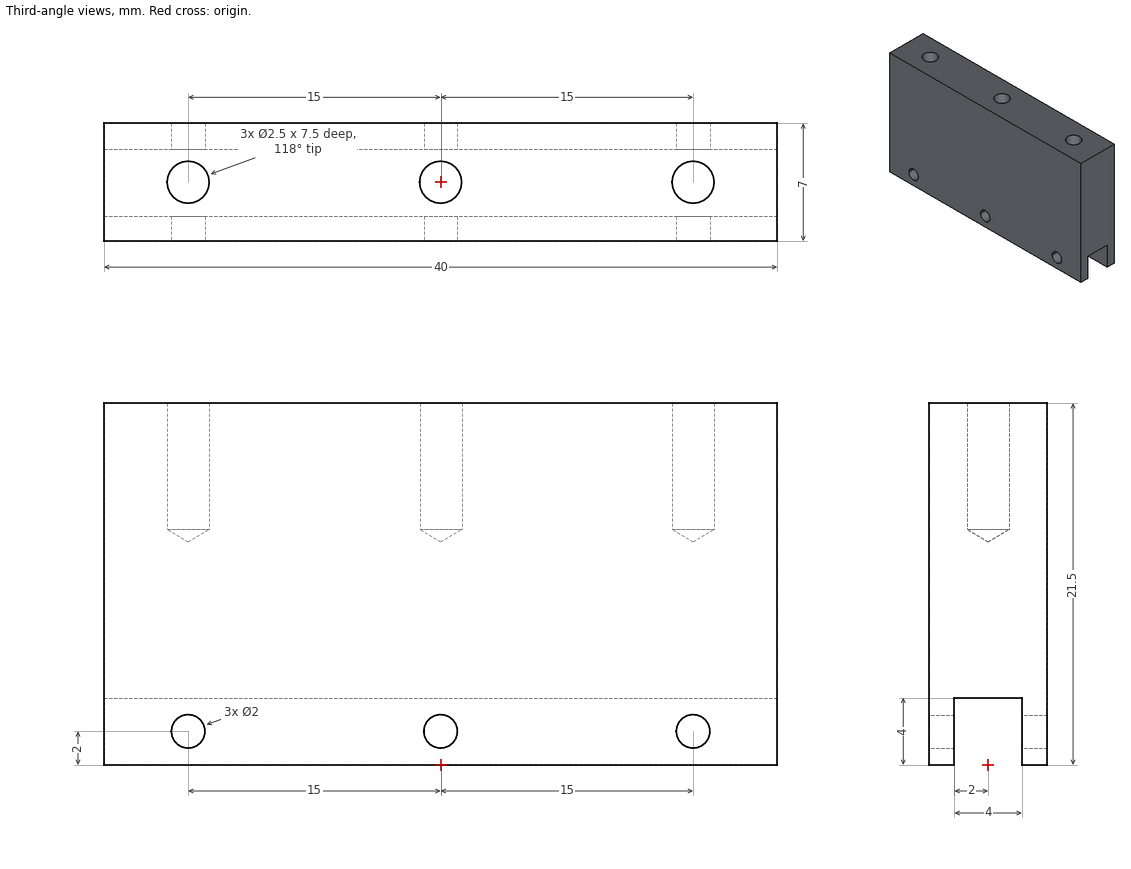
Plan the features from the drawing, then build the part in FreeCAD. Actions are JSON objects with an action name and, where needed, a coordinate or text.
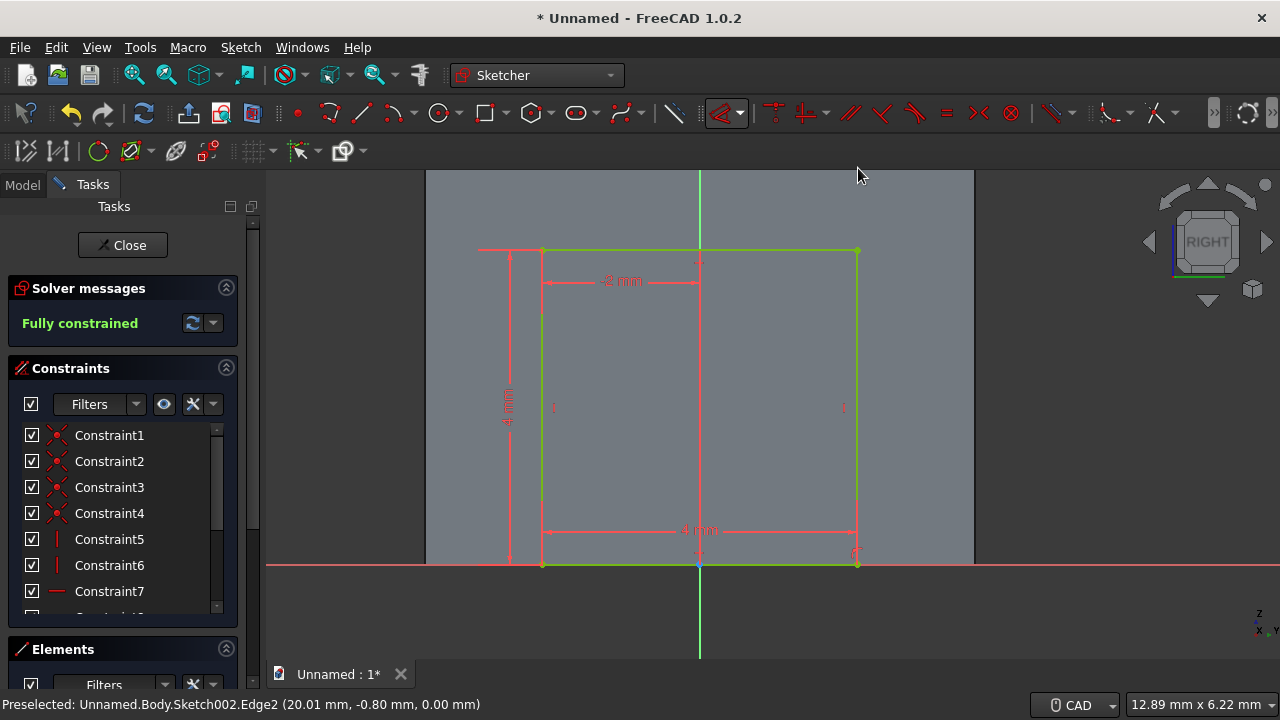
{"action": "left_click", "coordinate": [123, 245]}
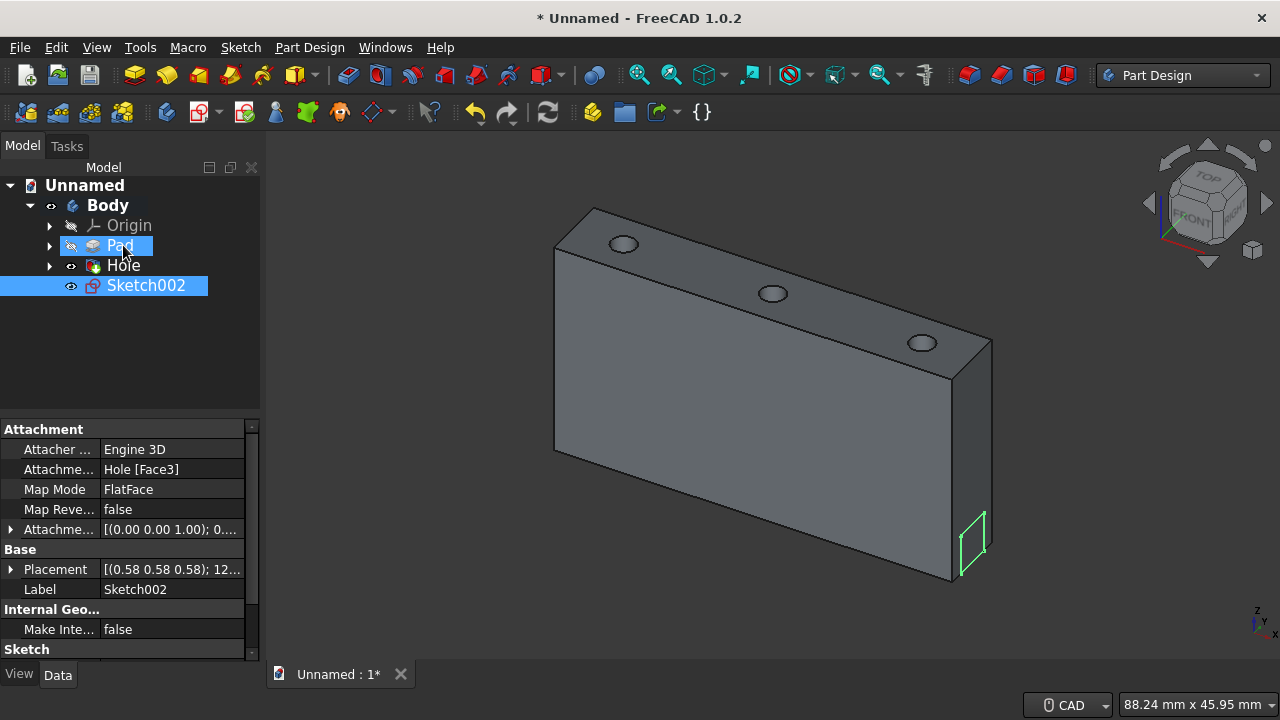
{"action": "left_click", "coordinate": [350, 76]}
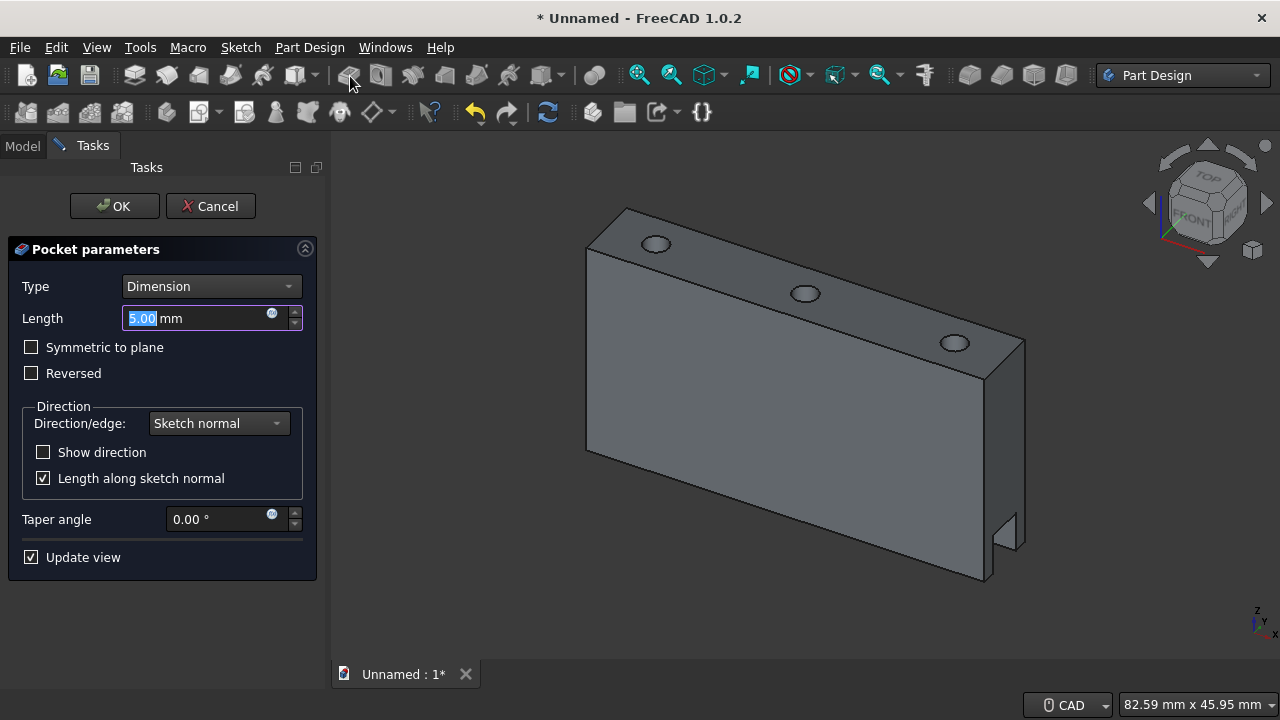
{"action": "left_click", "coordinate": [212, 286]}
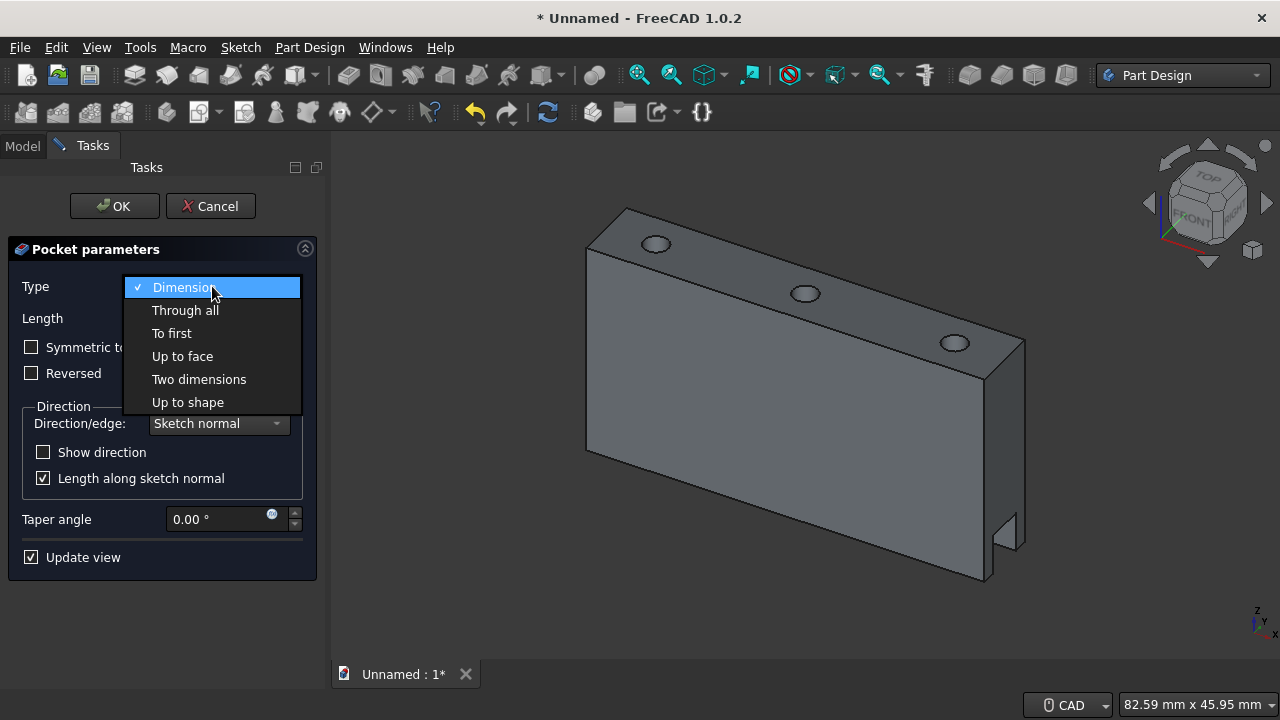
{"action": "left_click", "coordinate": [212, 310]}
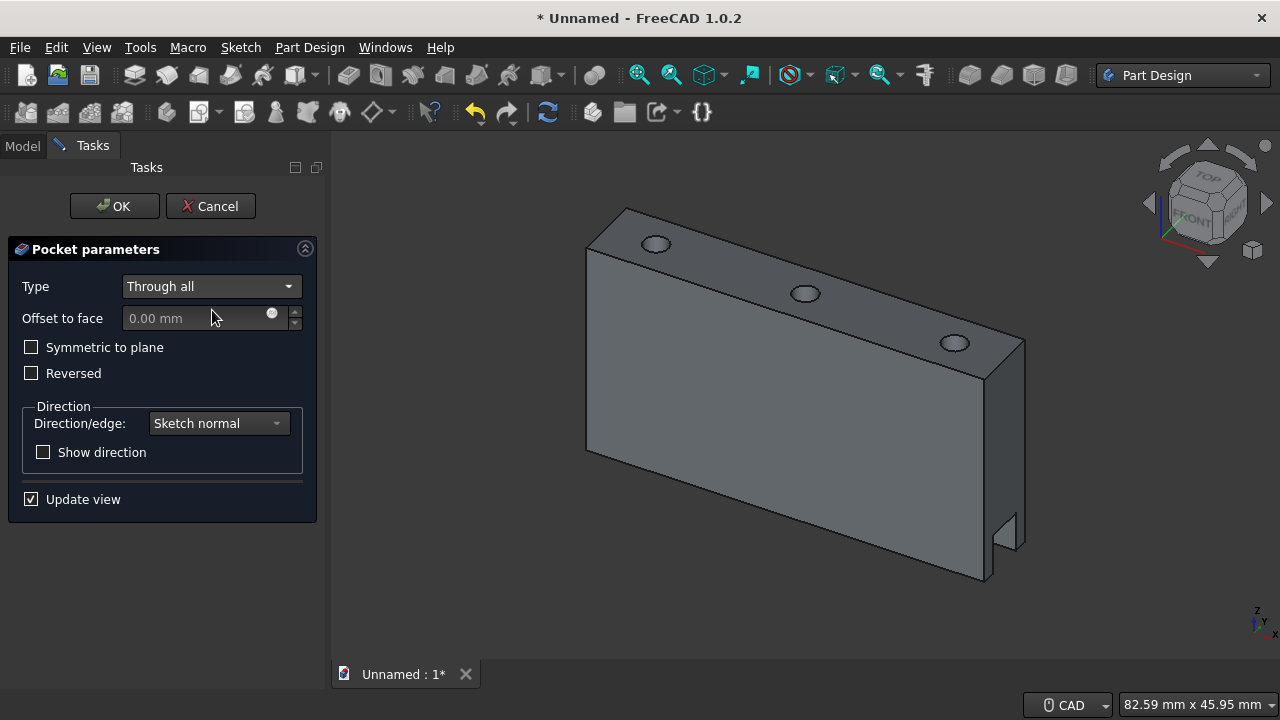
{"action": "left_click", "coordinate": [115, 206]}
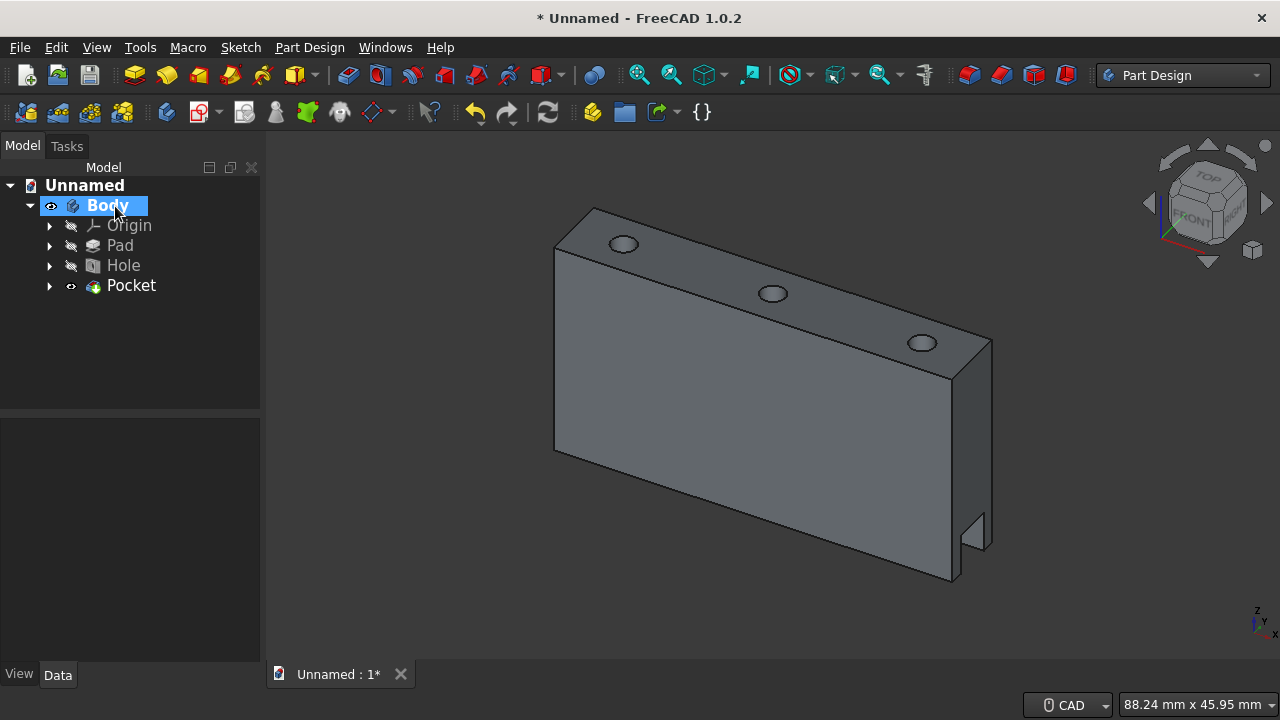
{"action": "key", "text": "4"}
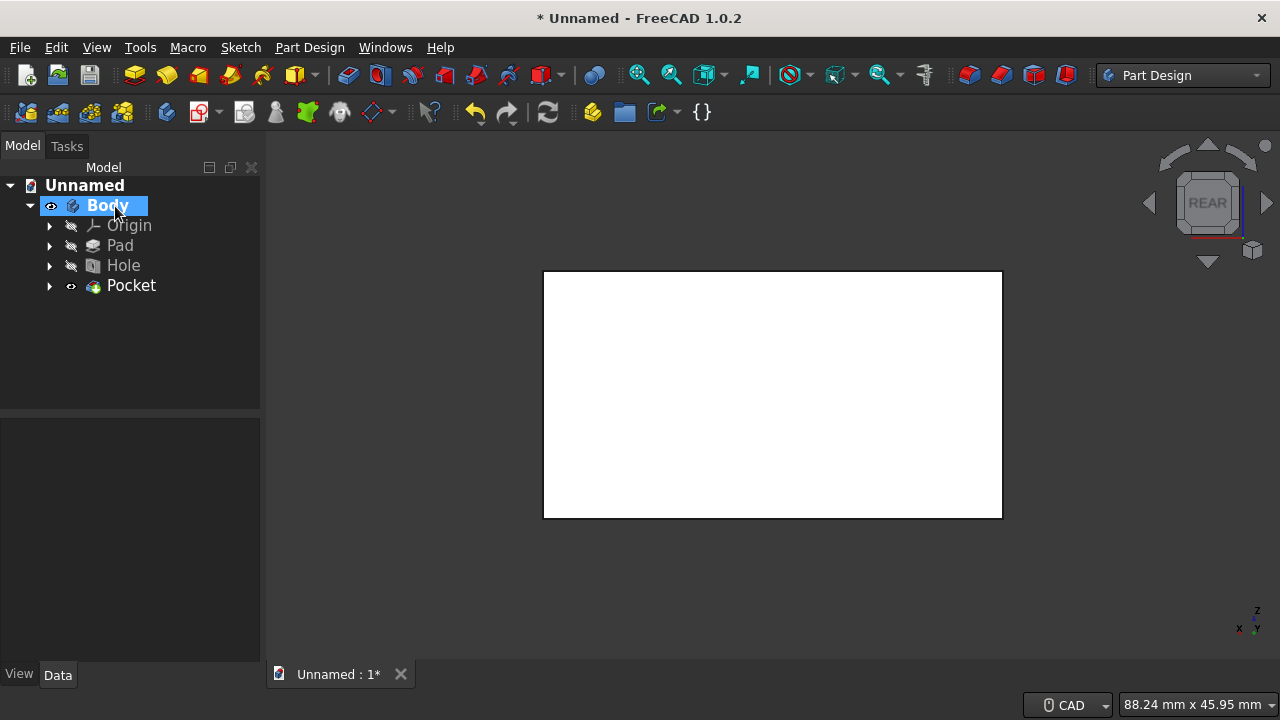
{"action": "left_click", "coordinate": [707, 394]}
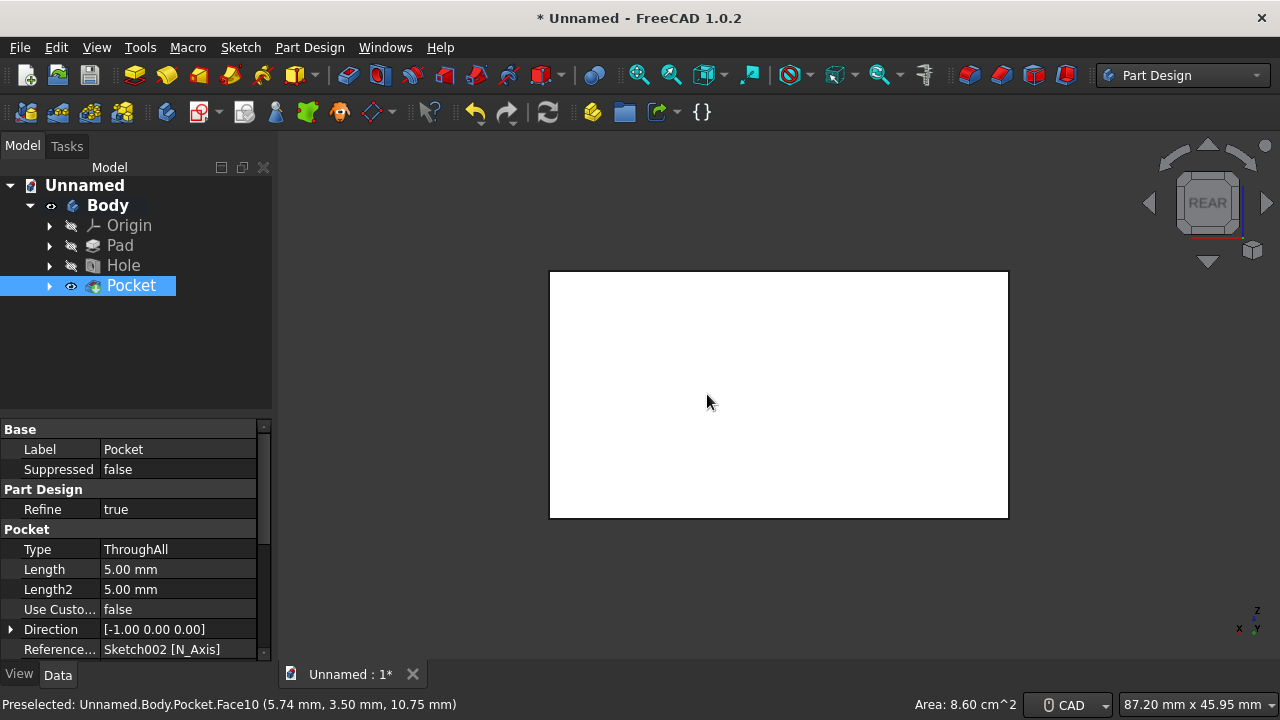
{"action": "left_click", "coordinate": [200, 112]}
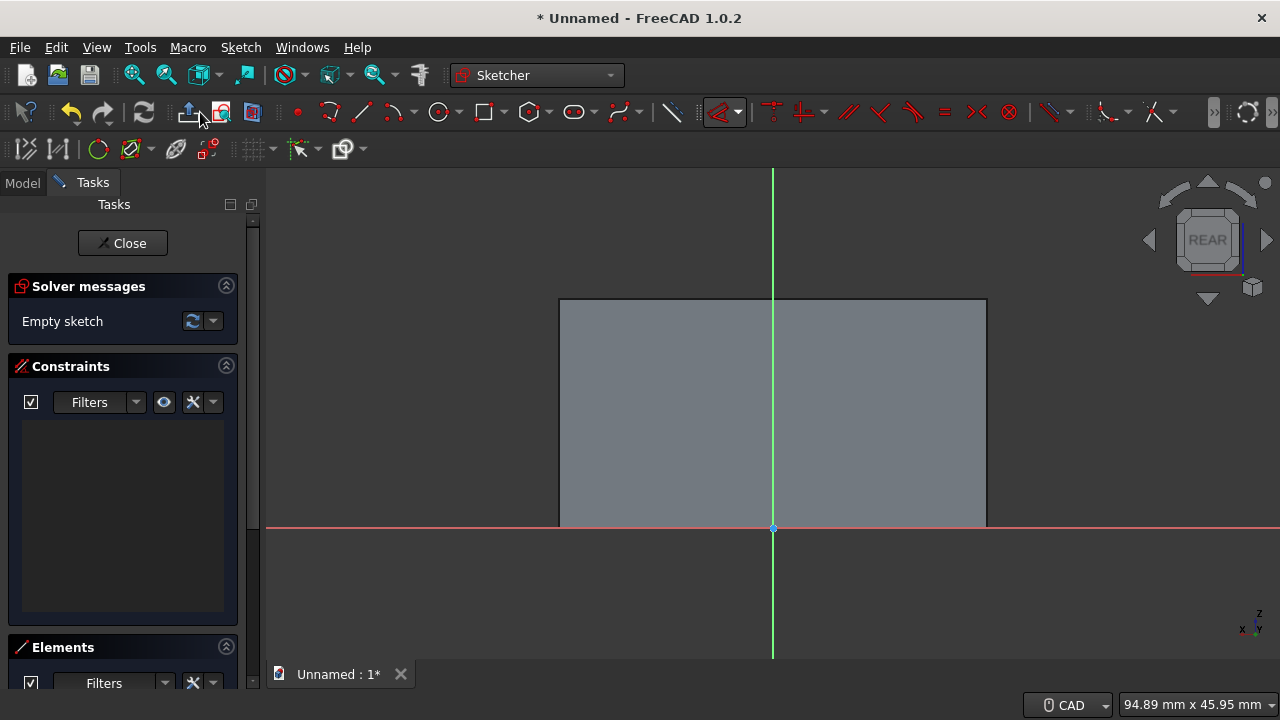
{"action": "scroll", "coordinate": [856, 631], "scroll_direction": "up", "scroll_amount": 3}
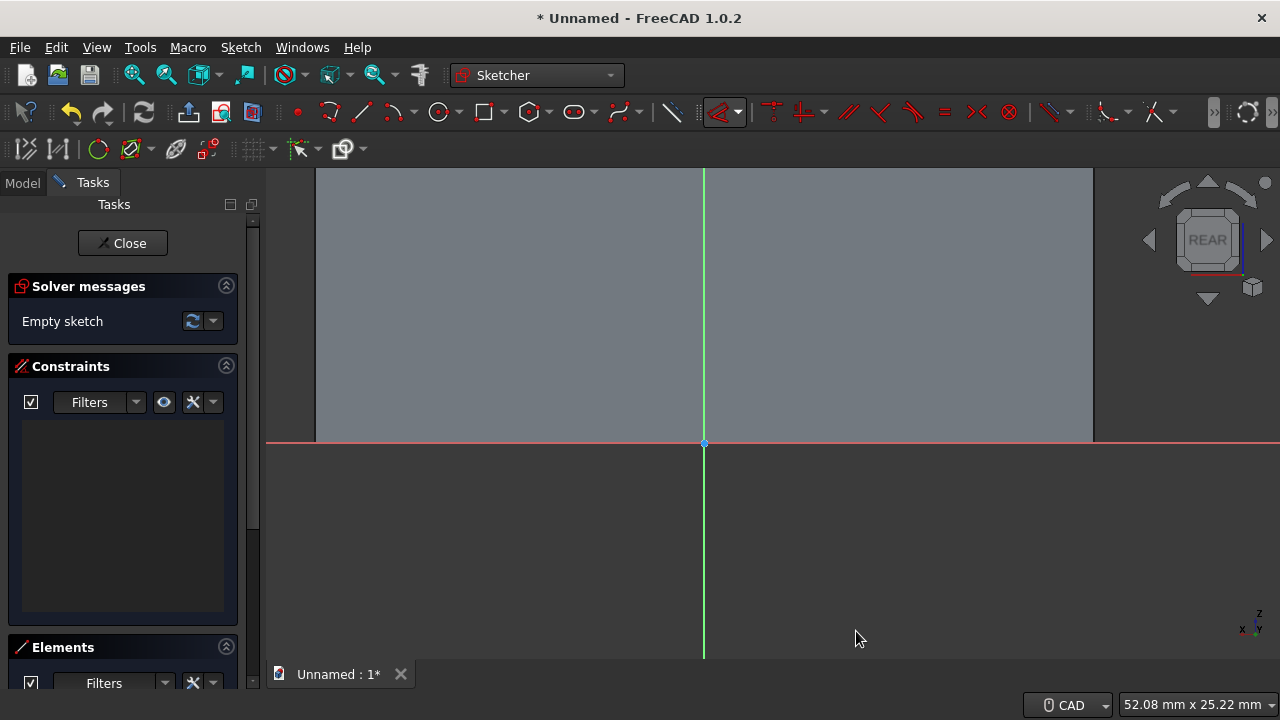
{"action": "left_click", "coordinate": [440, 112]}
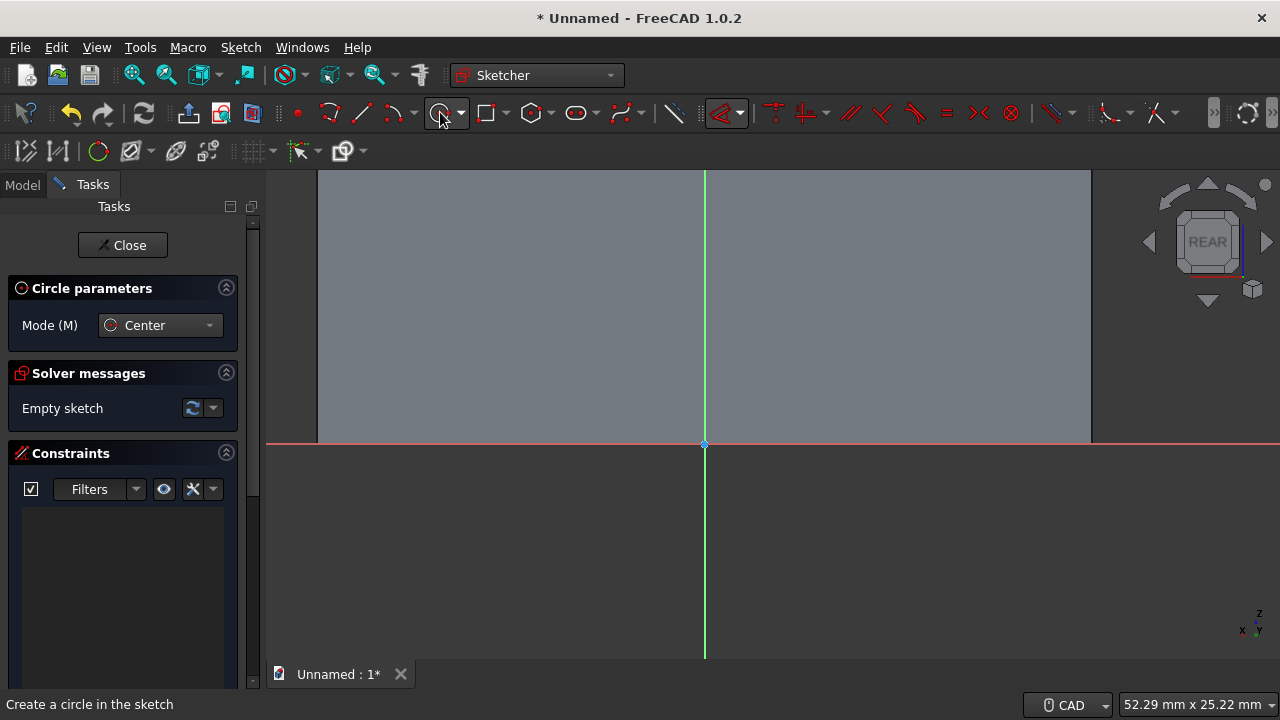
{"action": "left_click", "coordinate": [995, 405]}
{"action": "left_click", "coordinate": [1009, 392]}